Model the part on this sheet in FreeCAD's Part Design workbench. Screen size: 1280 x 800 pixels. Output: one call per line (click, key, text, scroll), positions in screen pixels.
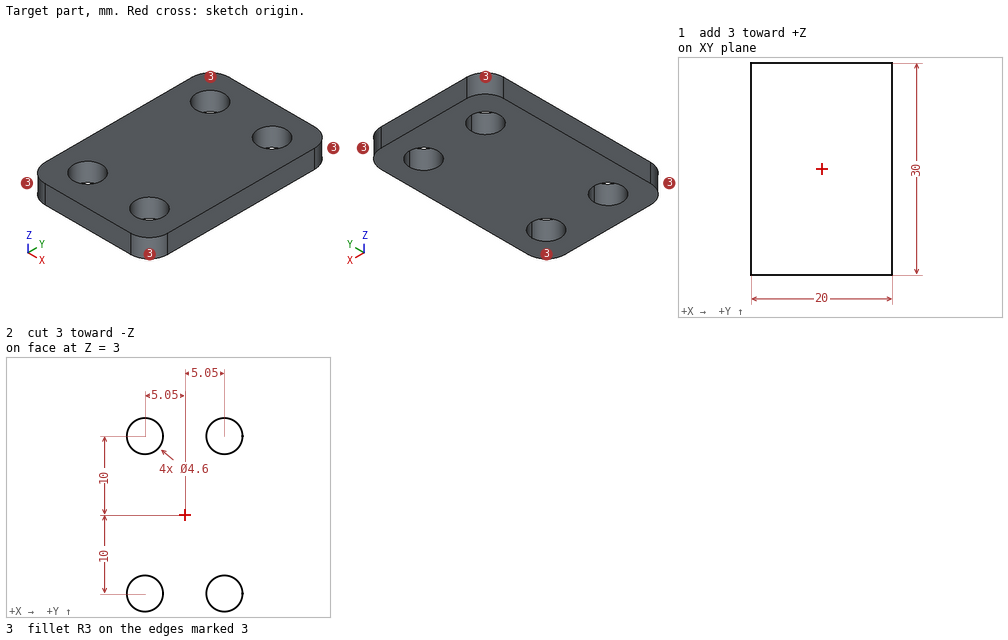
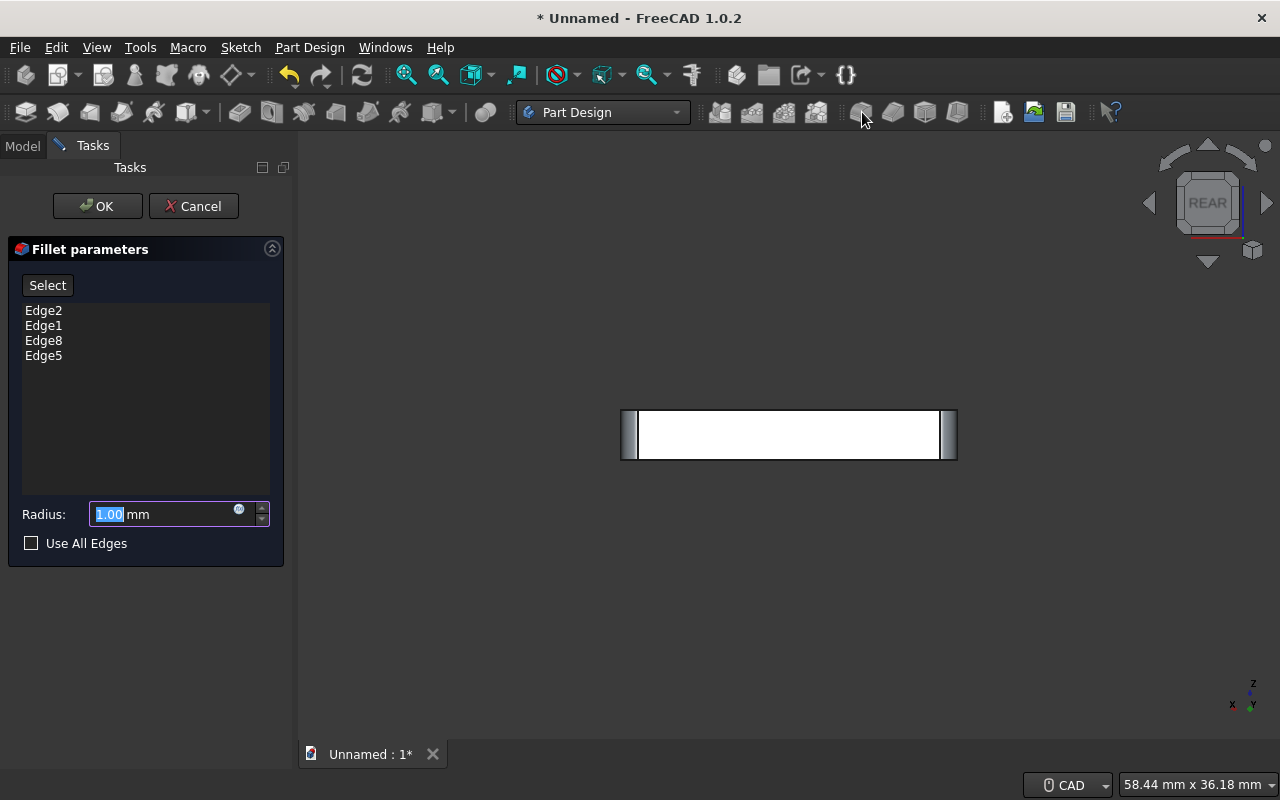
text(3)
key(Tab)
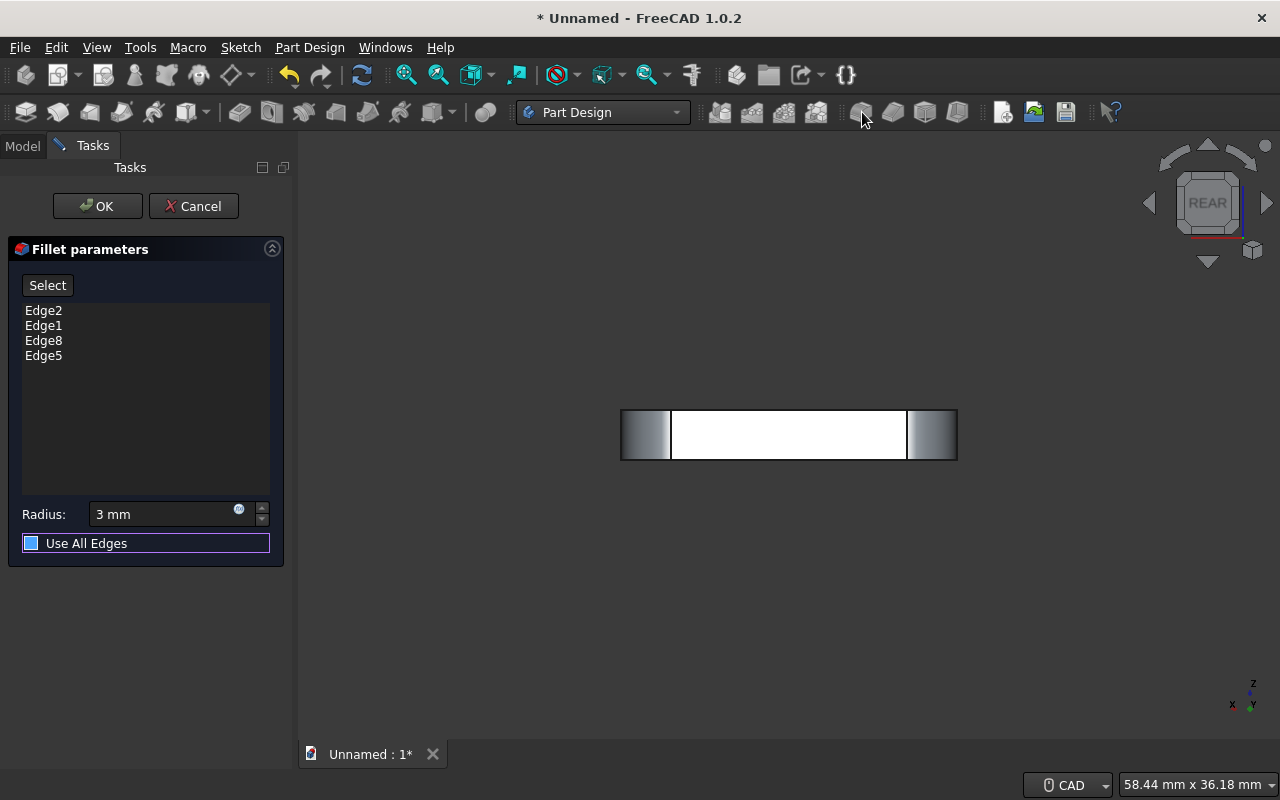
click(98, 206)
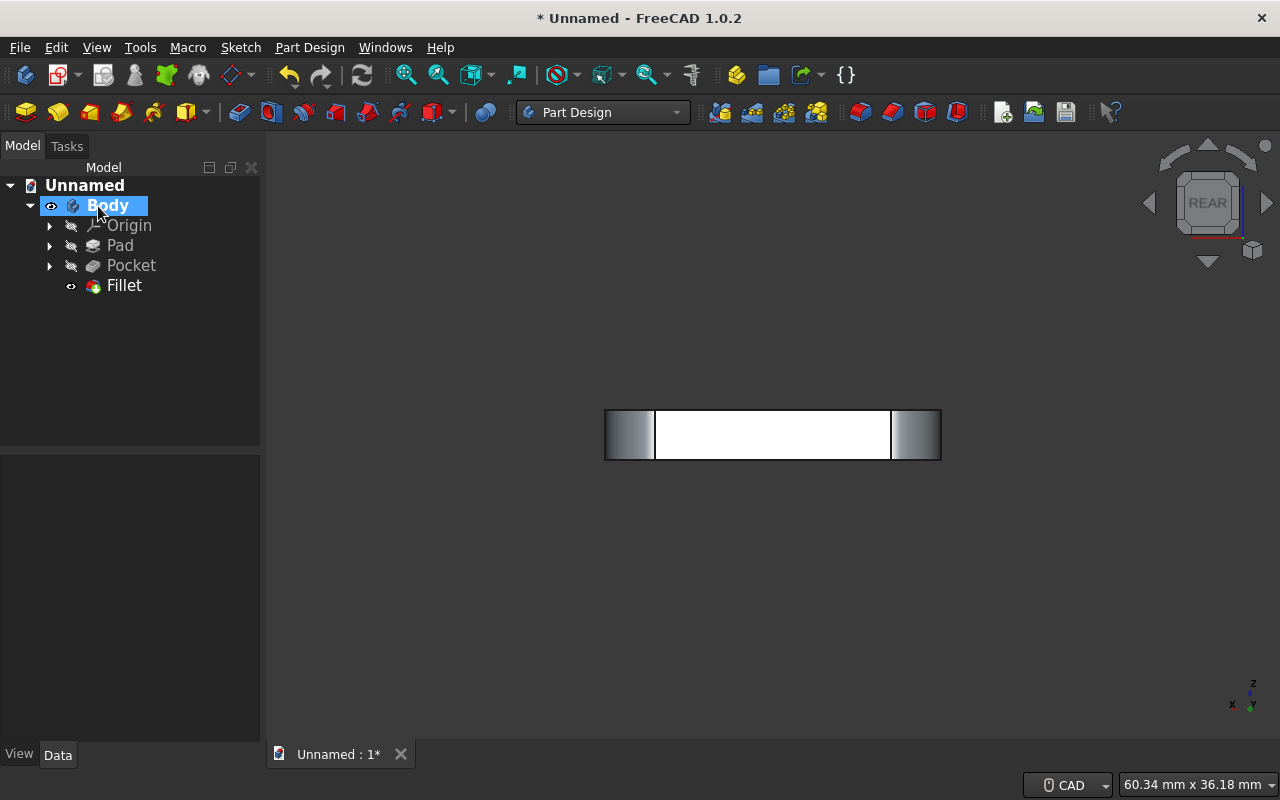
key(0)